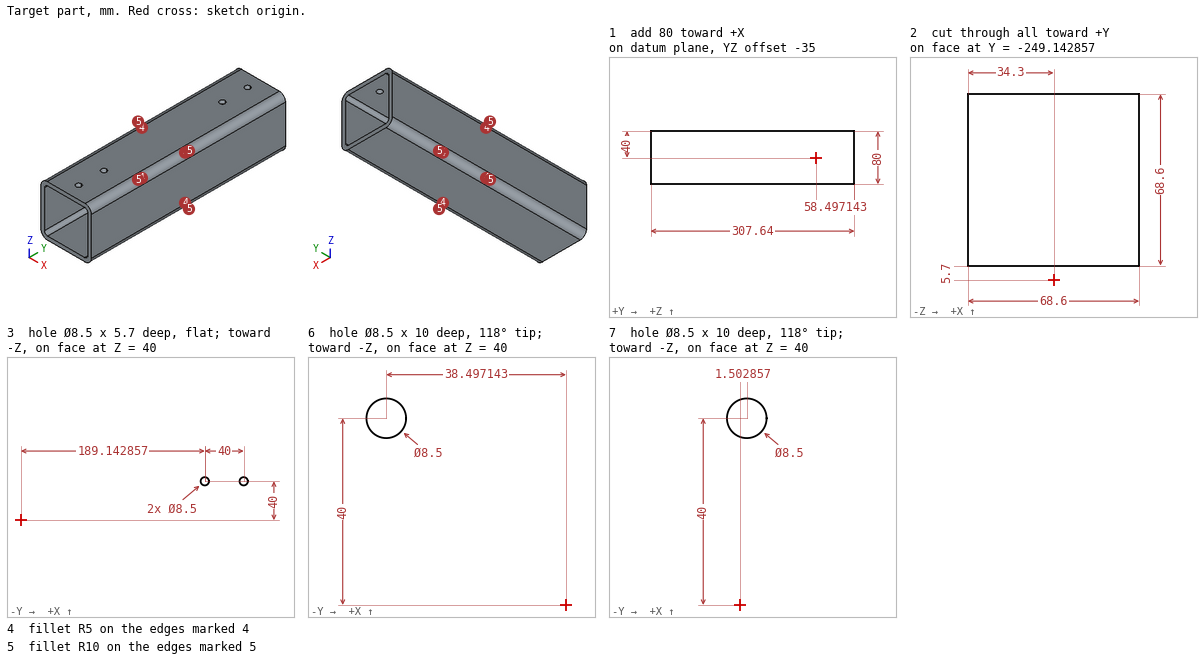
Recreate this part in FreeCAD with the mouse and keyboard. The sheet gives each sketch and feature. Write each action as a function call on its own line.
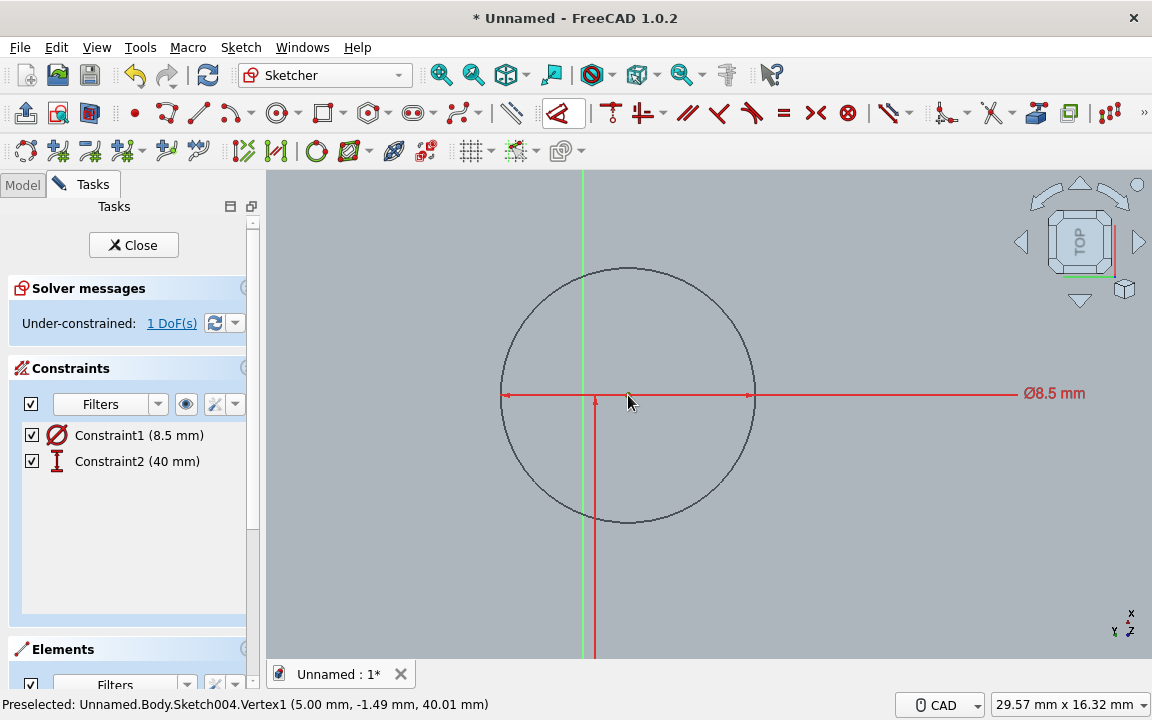
key(l)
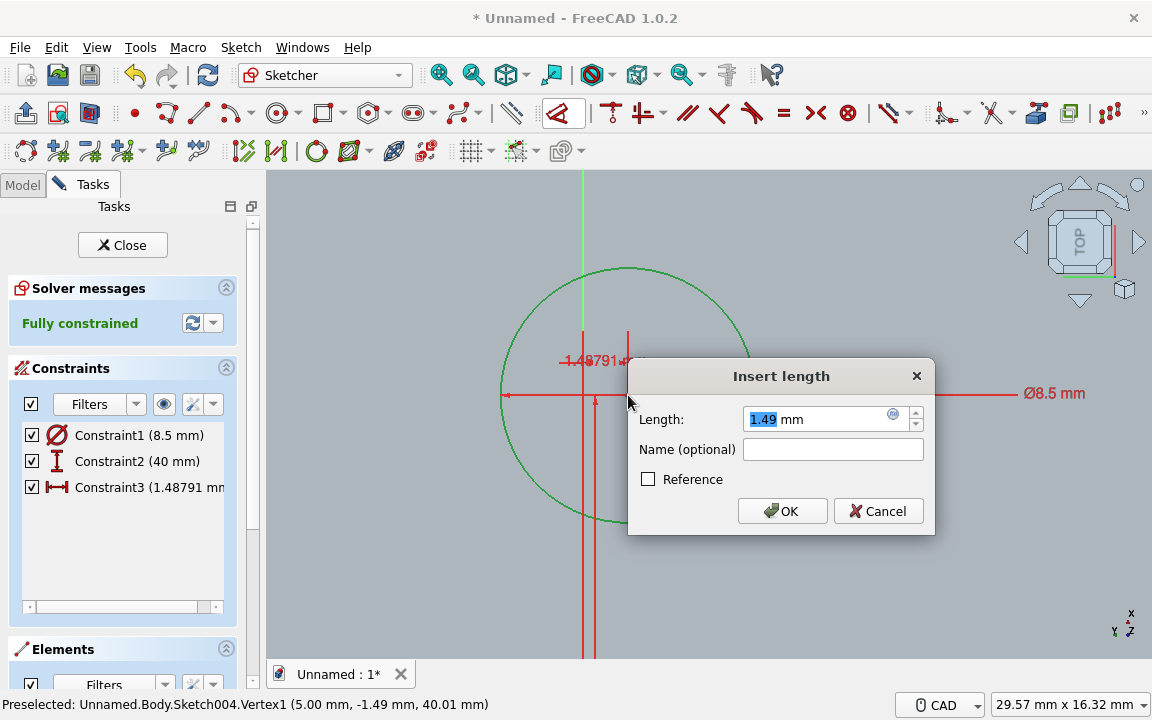
text(1.502857)
key(Return)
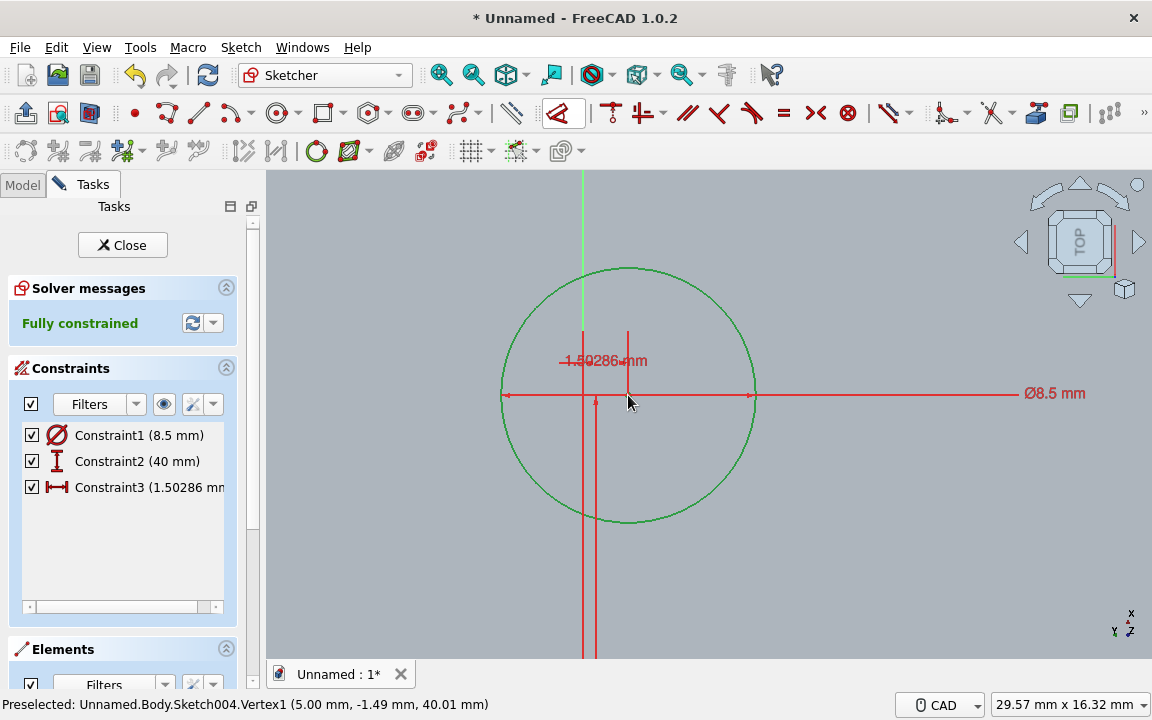
click(123, 245)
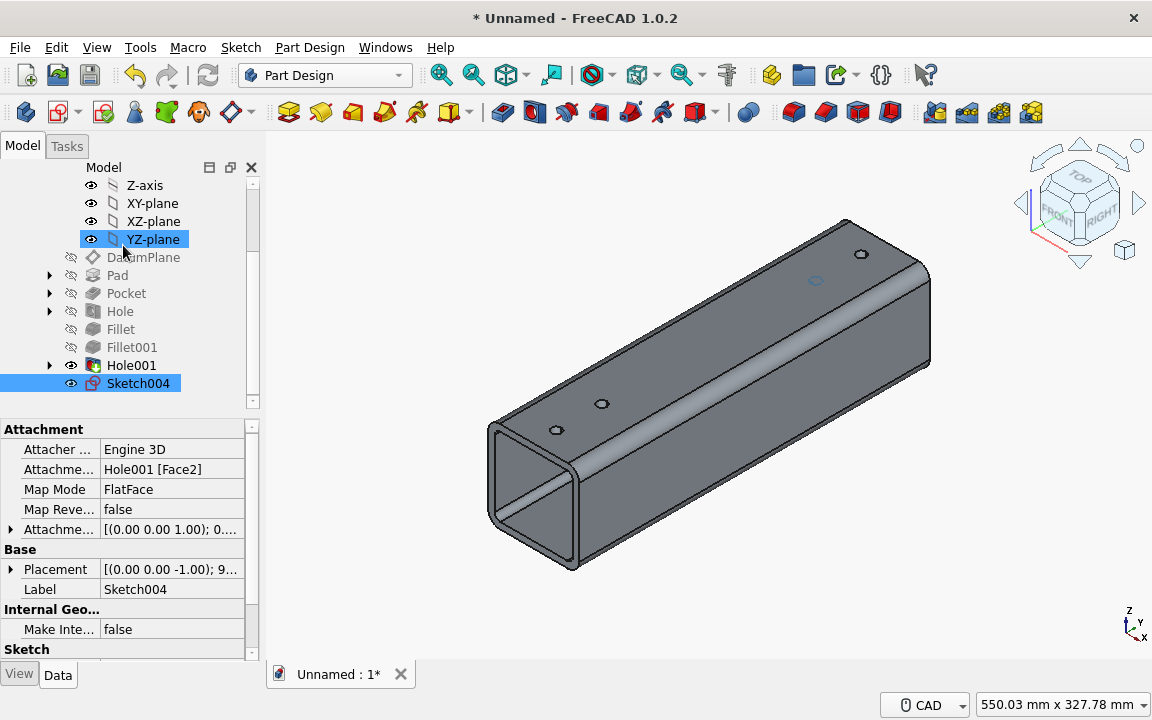
click(536, 112)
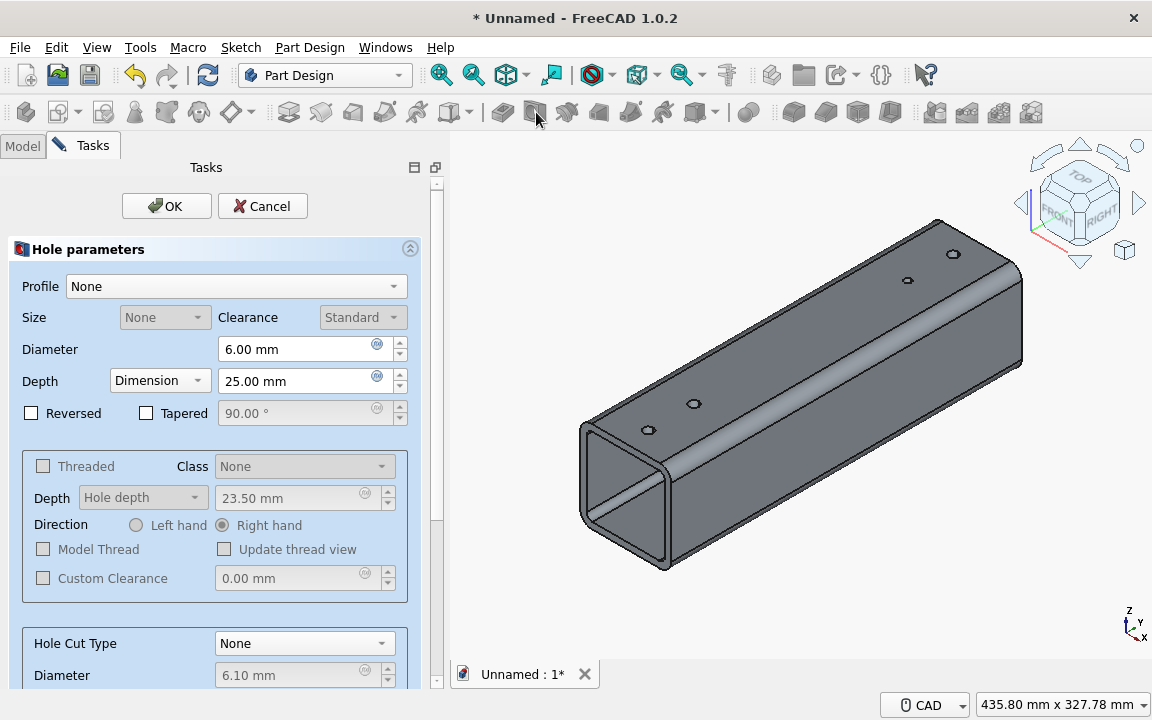
triple_click(305, 349)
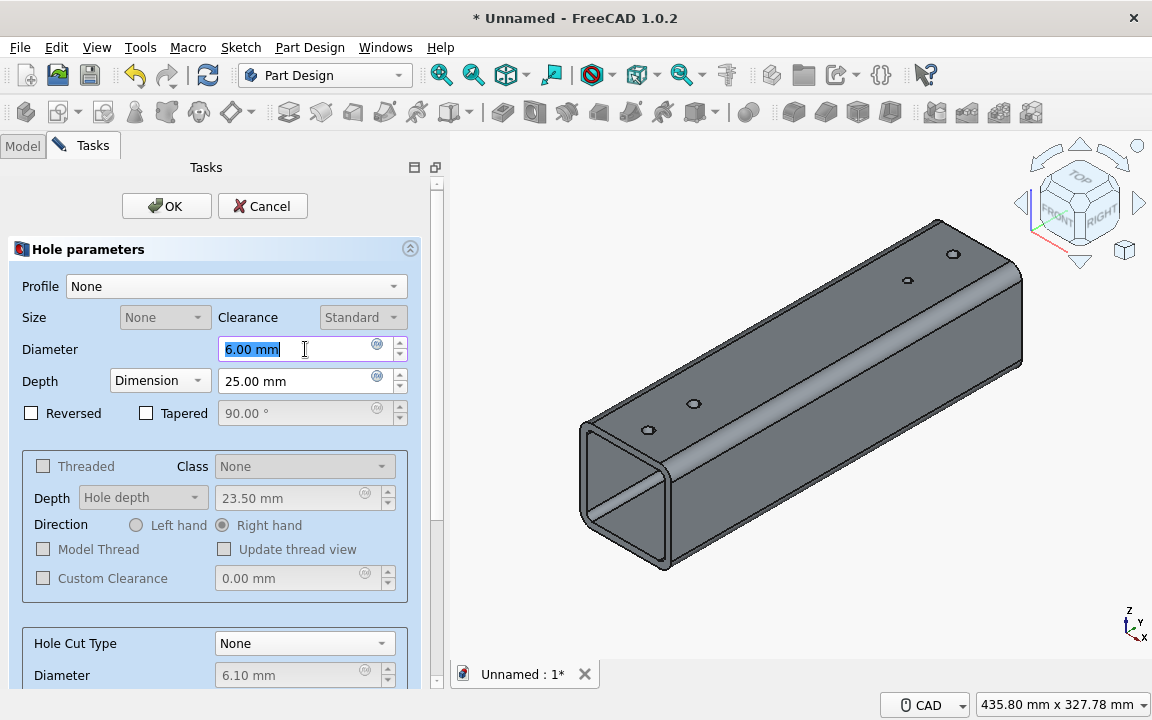
text(8.5)
key(Tab)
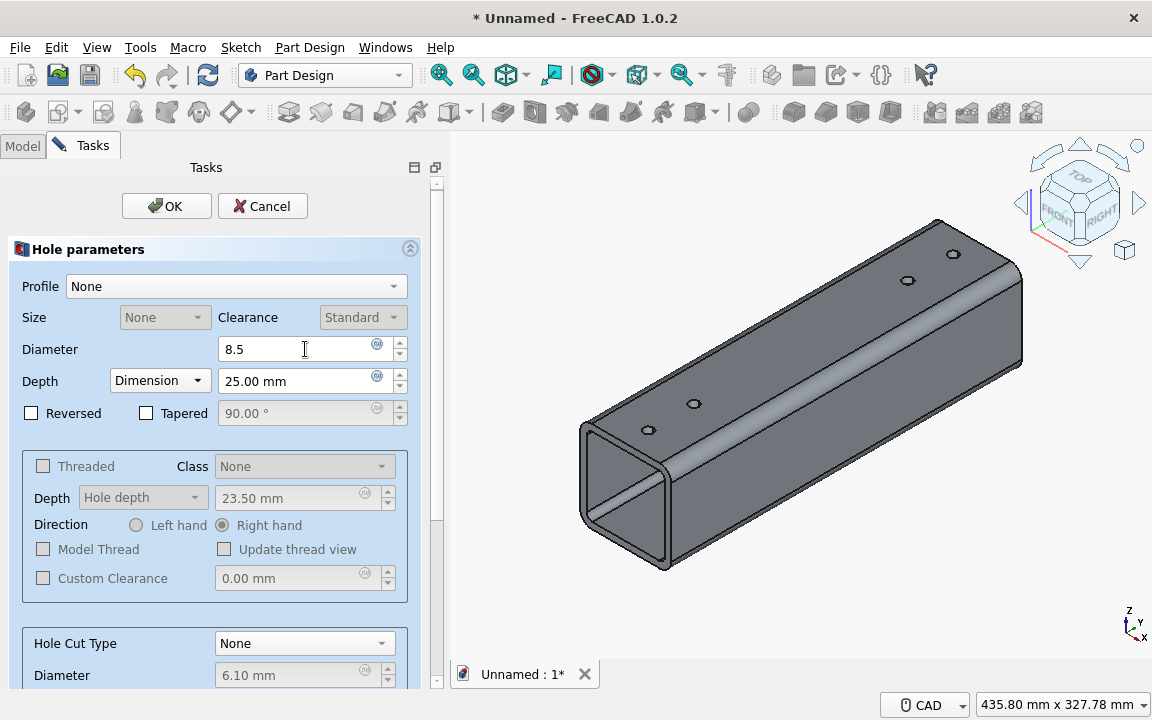
triple_click(305, 381)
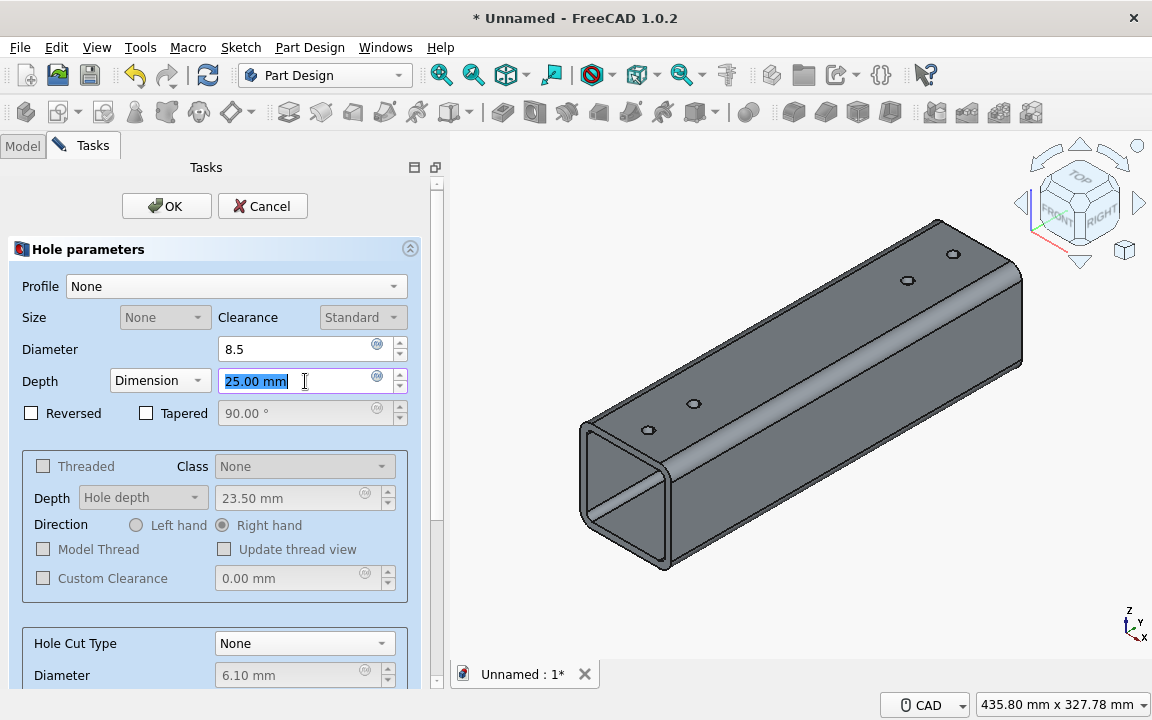
text(10)
key(Tab)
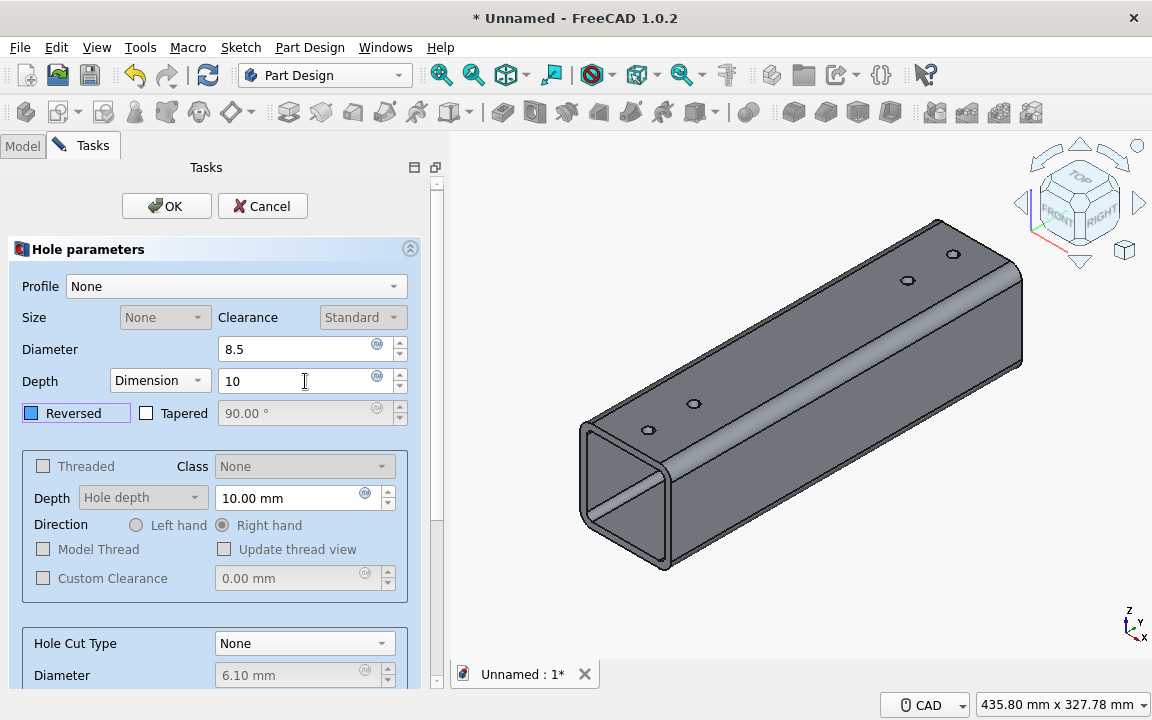
click(167, 206)